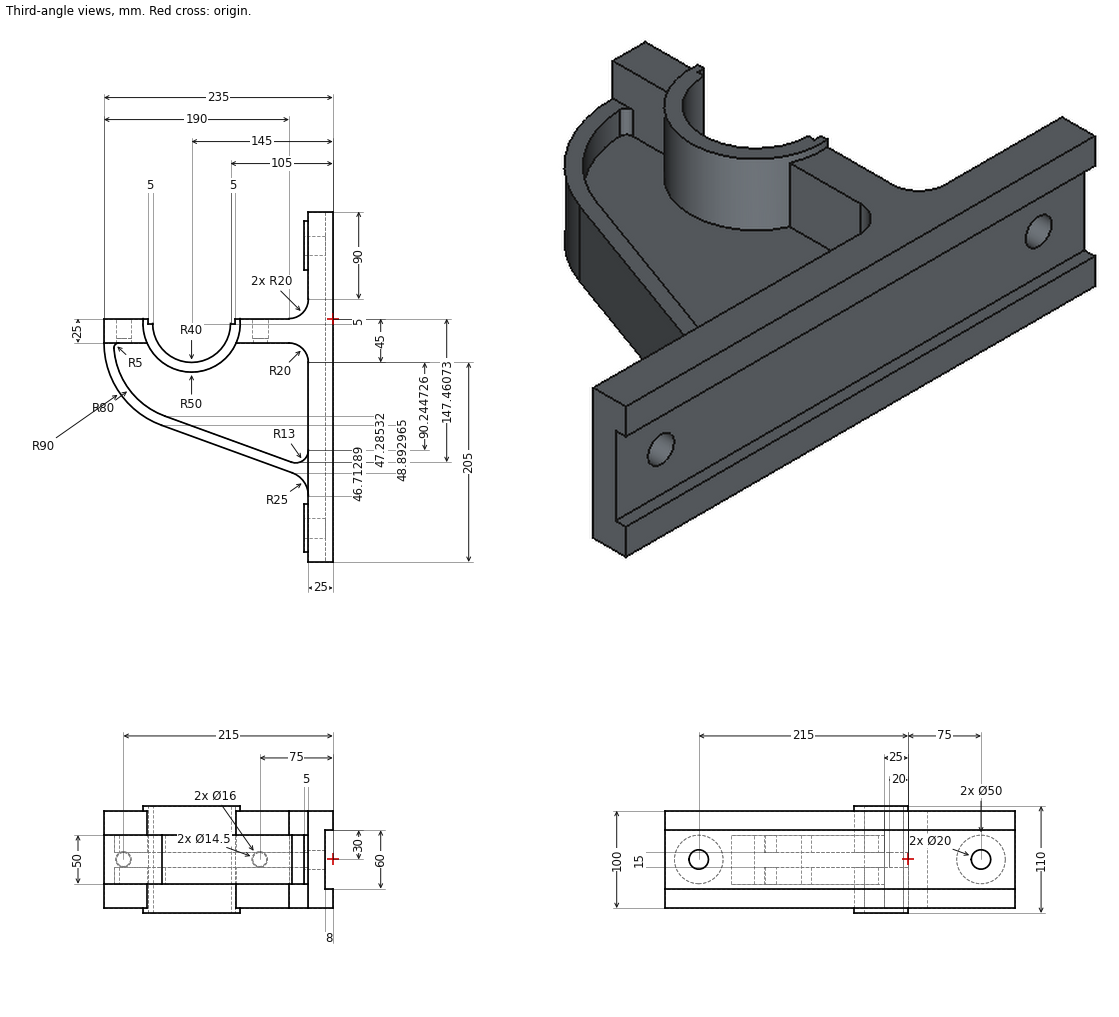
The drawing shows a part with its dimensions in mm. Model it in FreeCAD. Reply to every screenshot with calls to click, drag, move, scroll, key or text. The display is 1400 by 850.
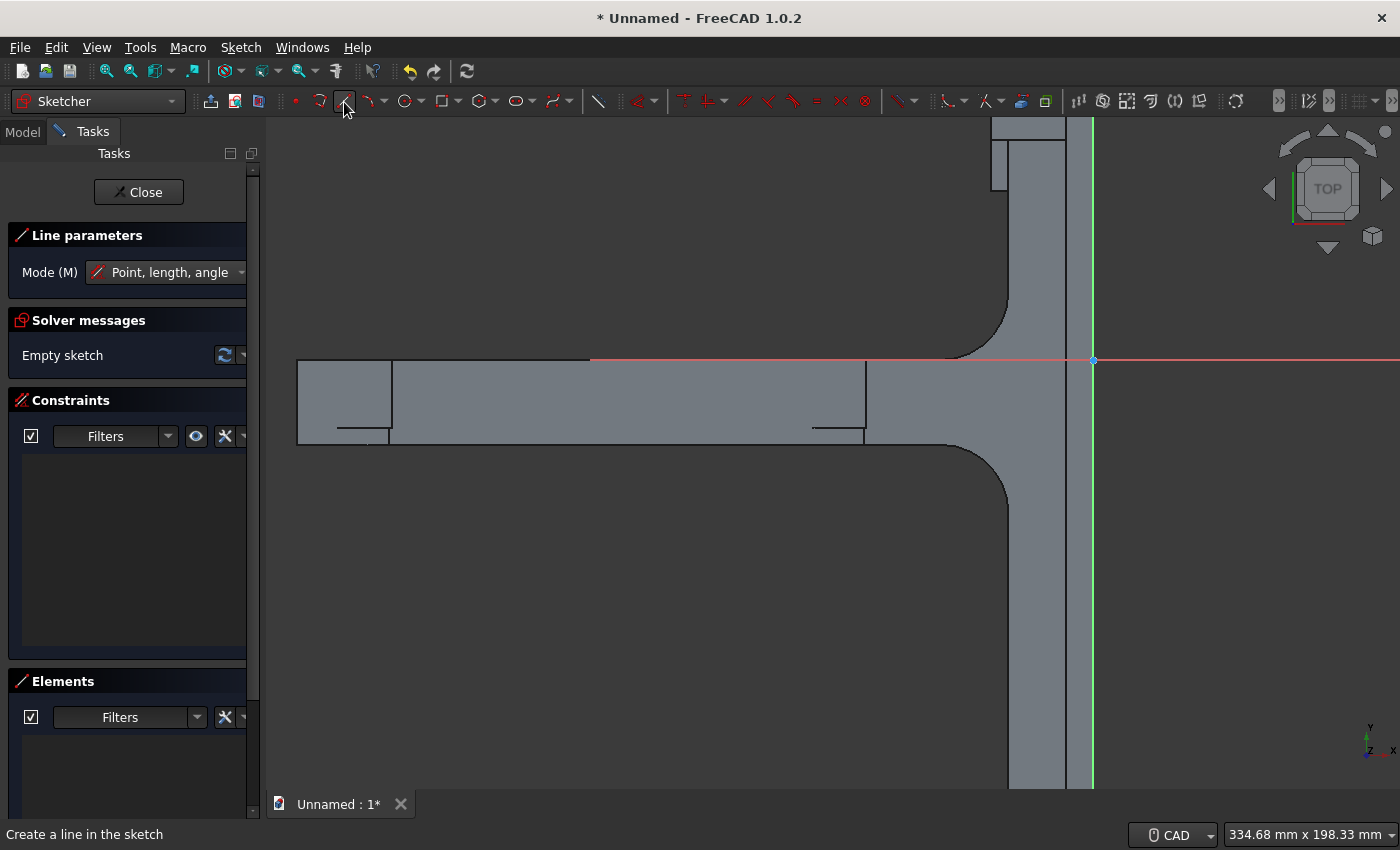
click(770, 360)
click(433, 369)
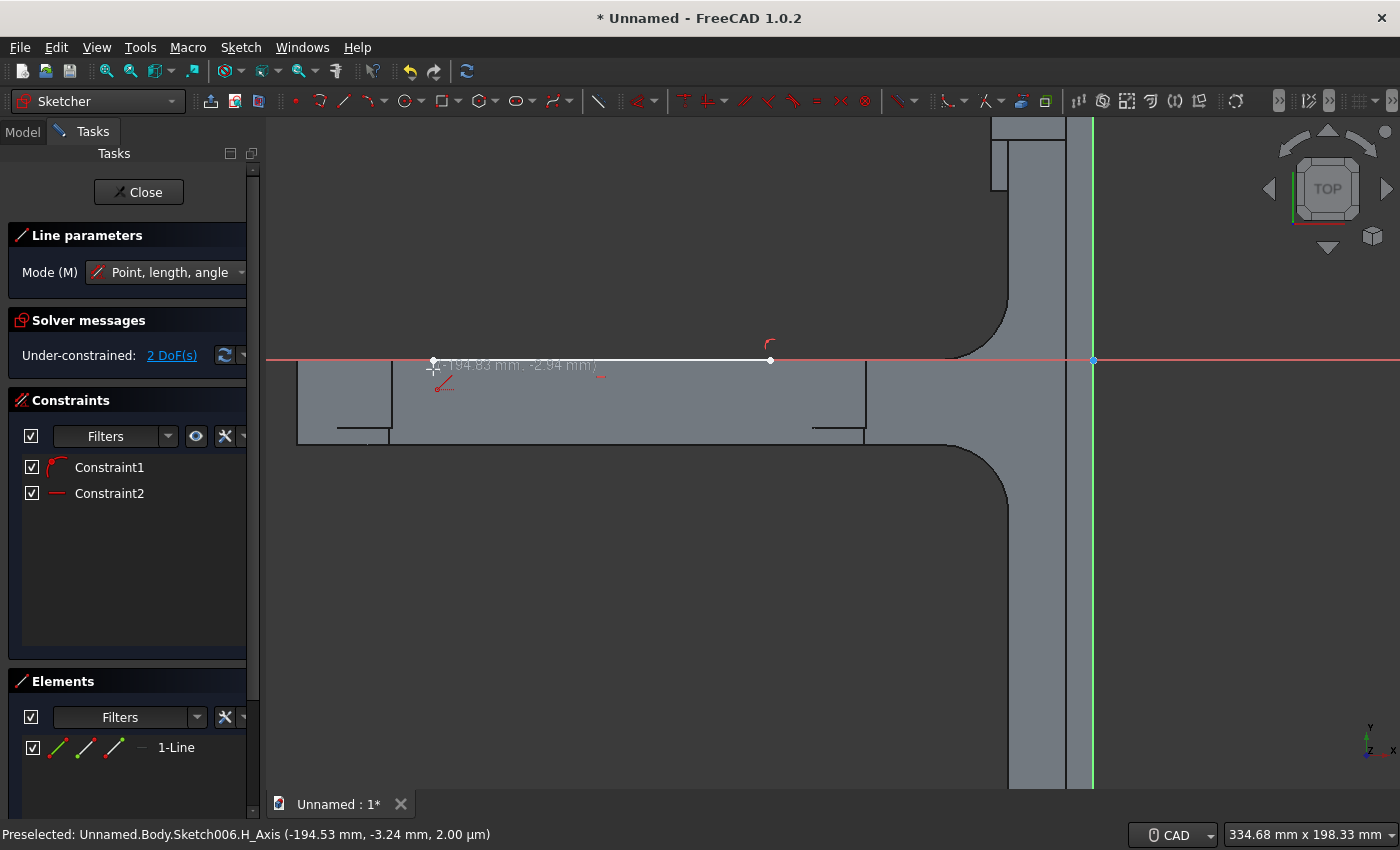
click(368, 102)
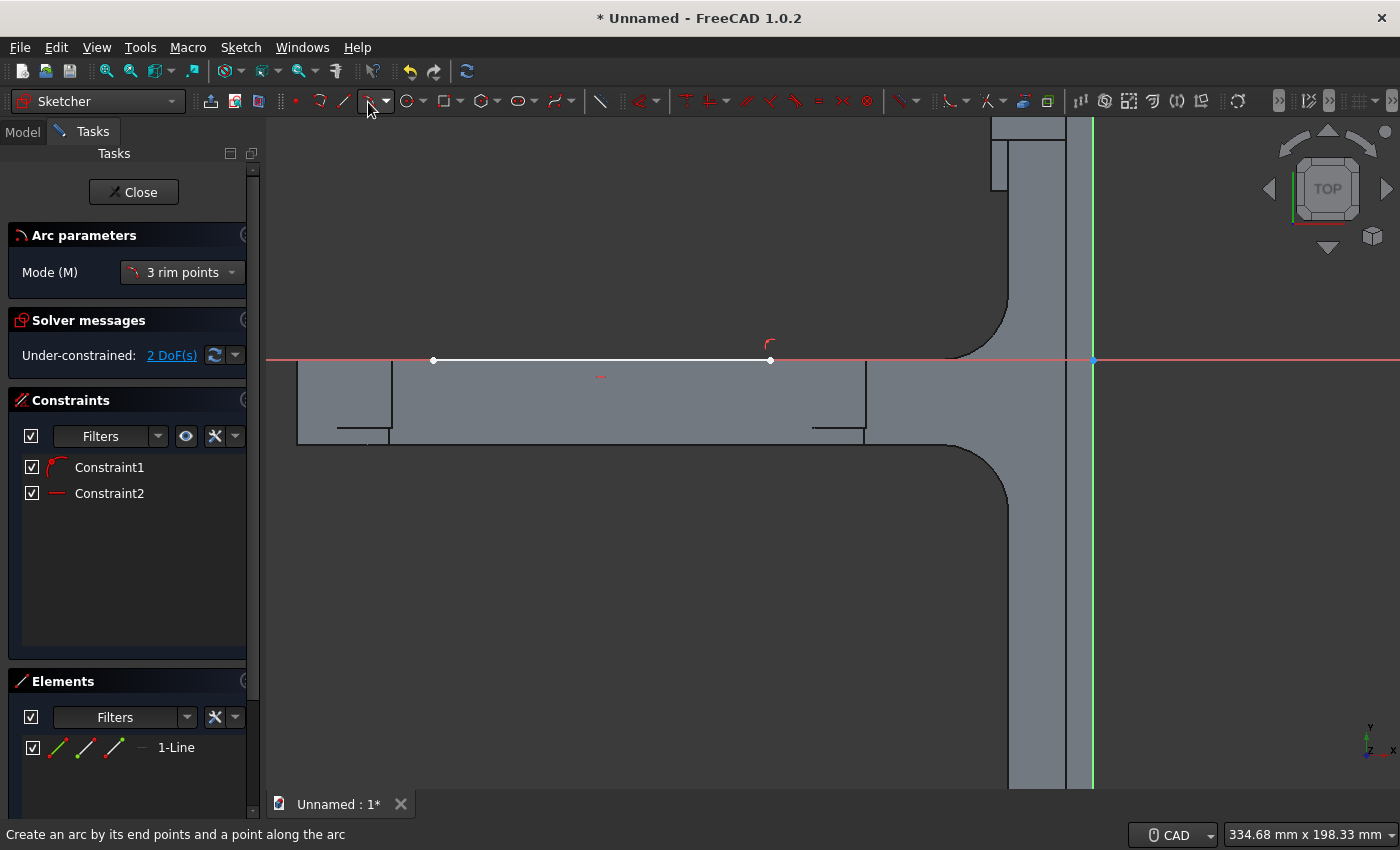
click(433, 360)
click(770, 360)
click(602, 546)
key(Escape)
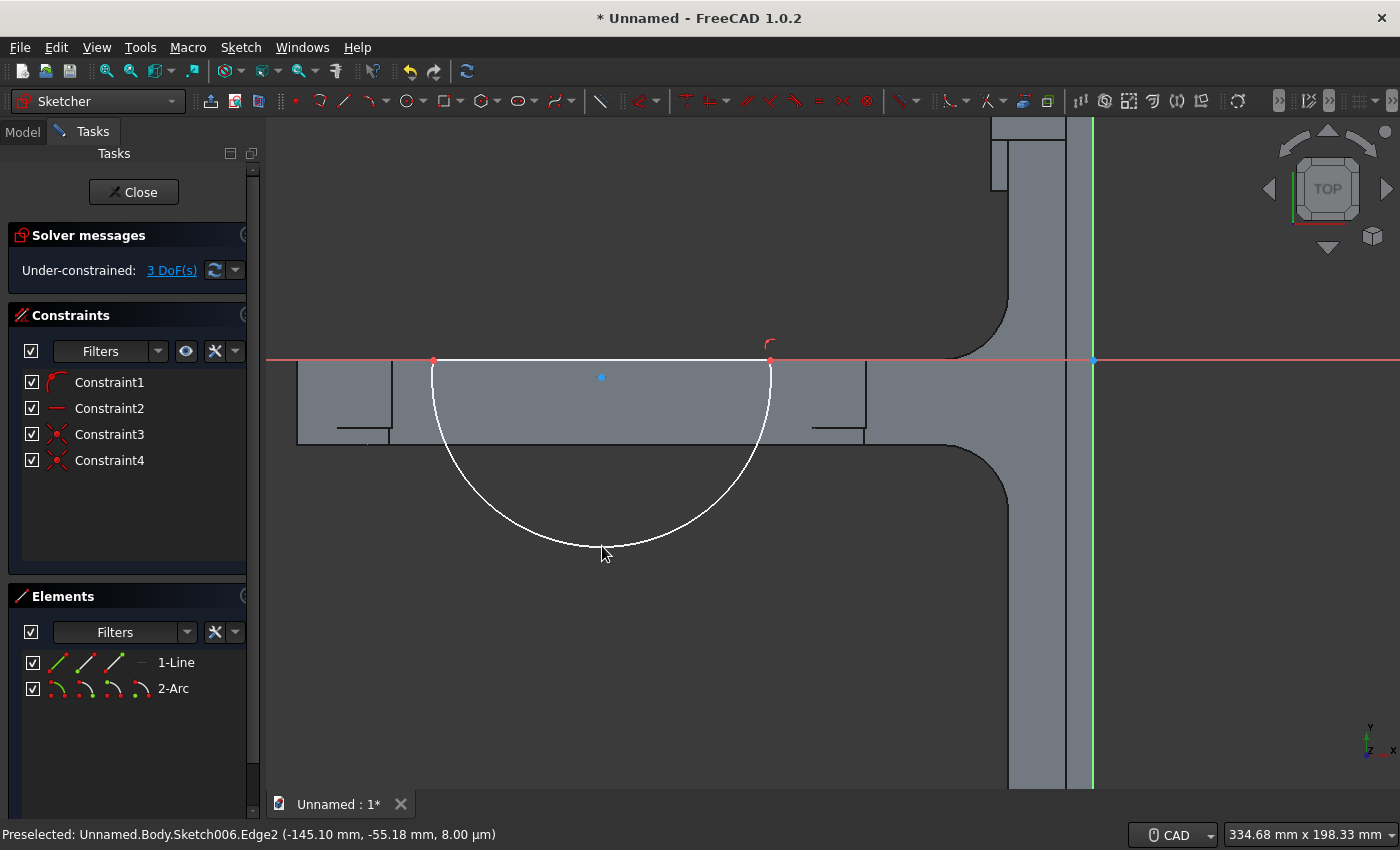
click(640, 102)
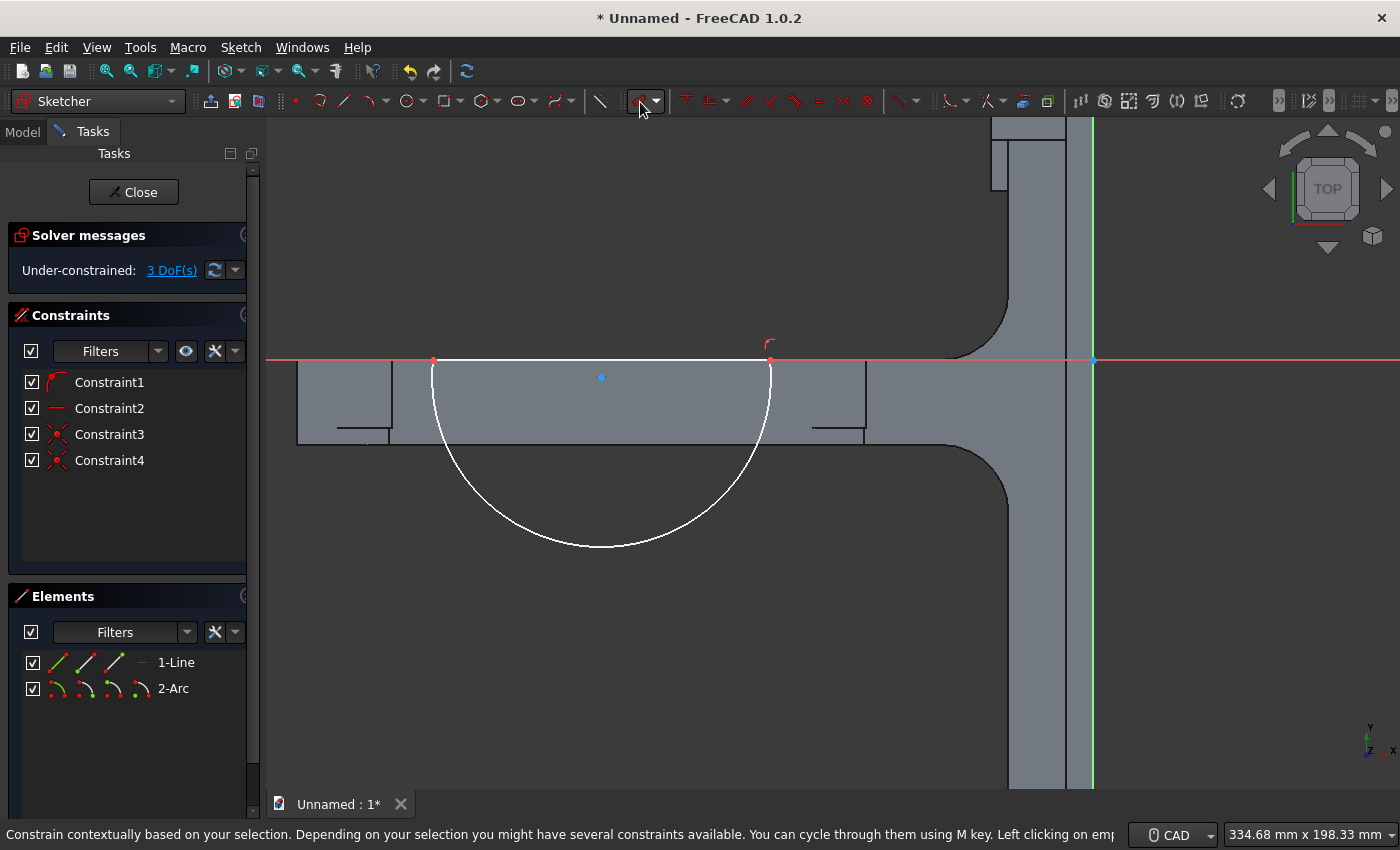
click(496, 510)
click(476, 535)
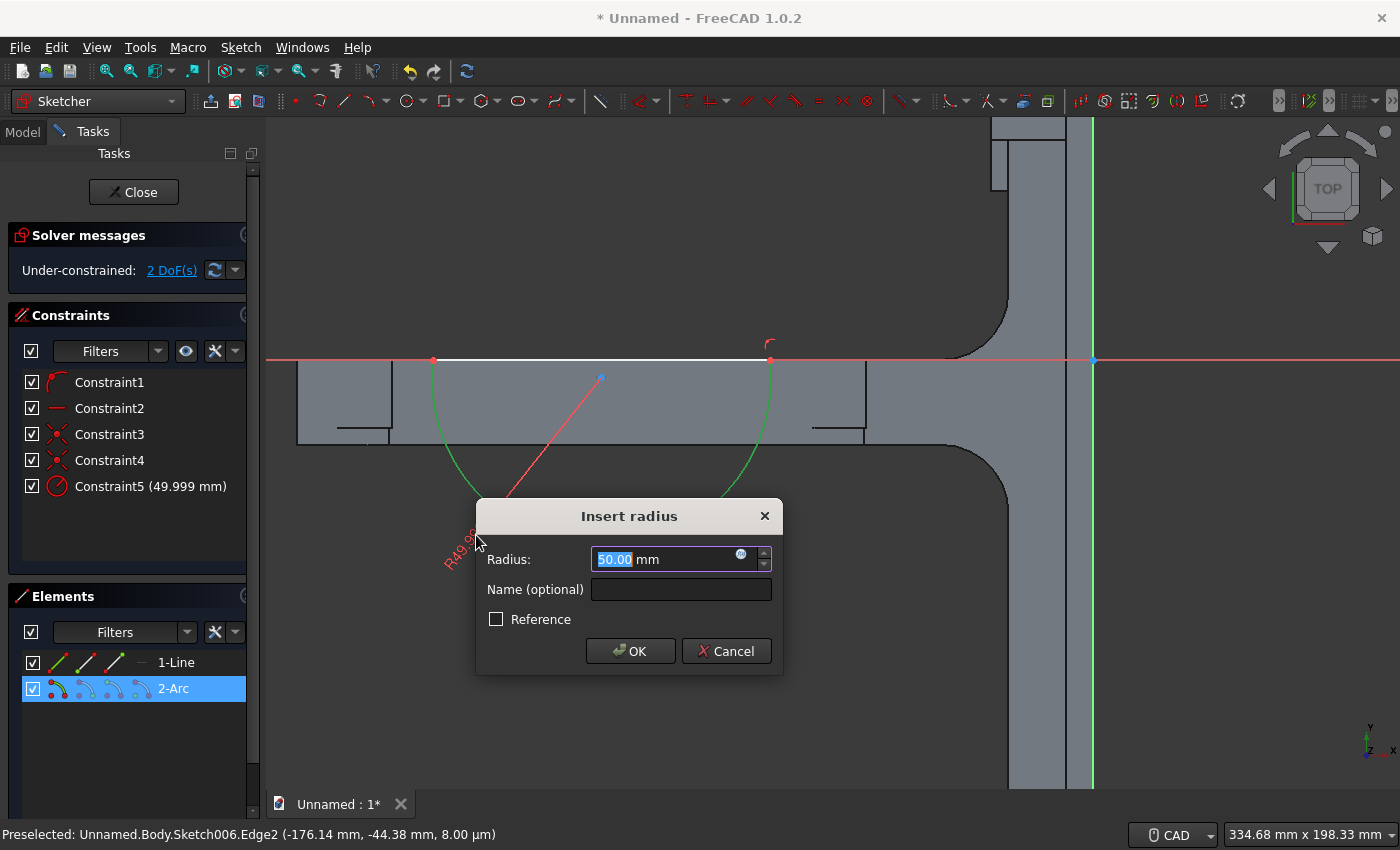
text(50)
key(Return)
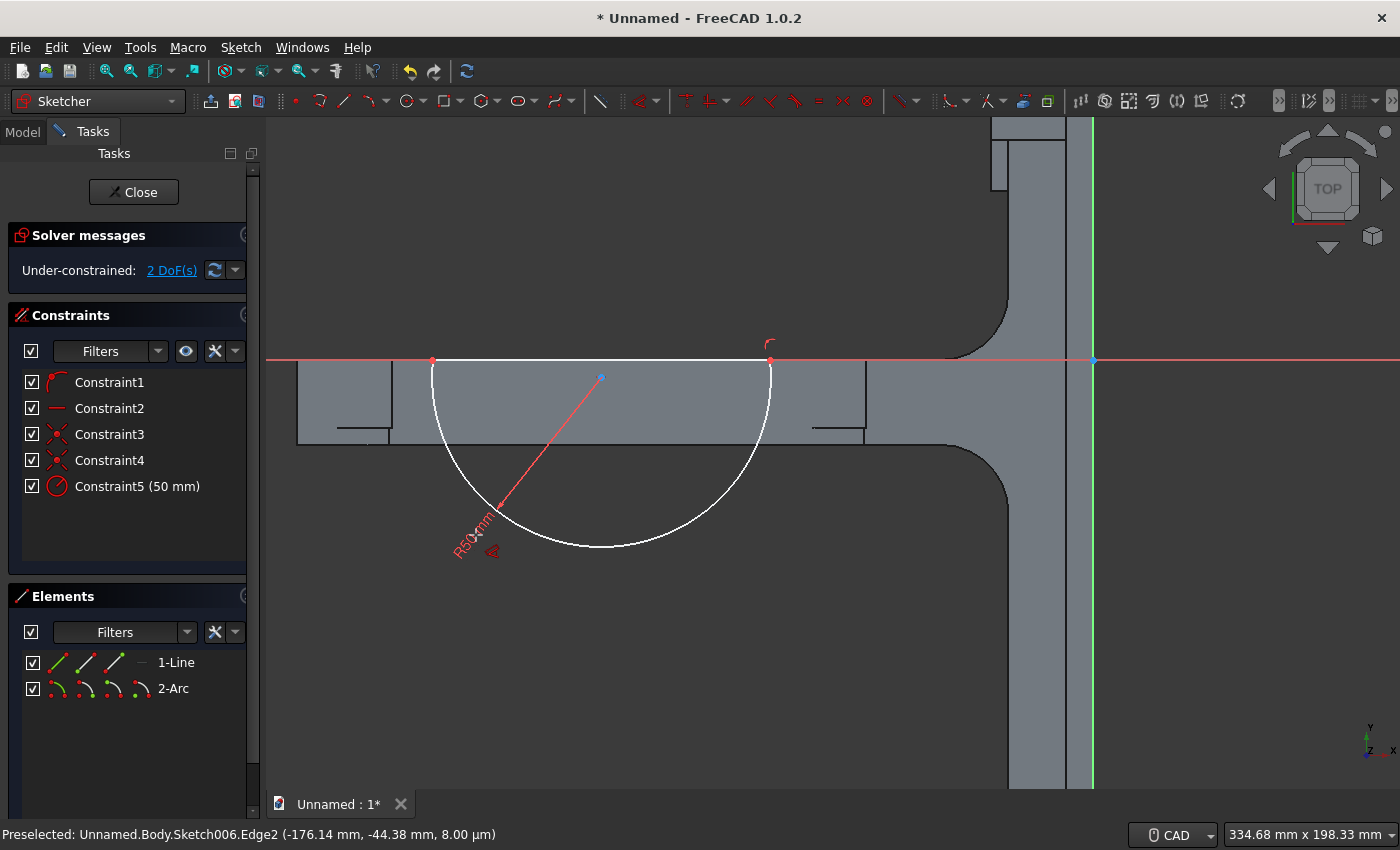
scroll(601, 378, up, 5)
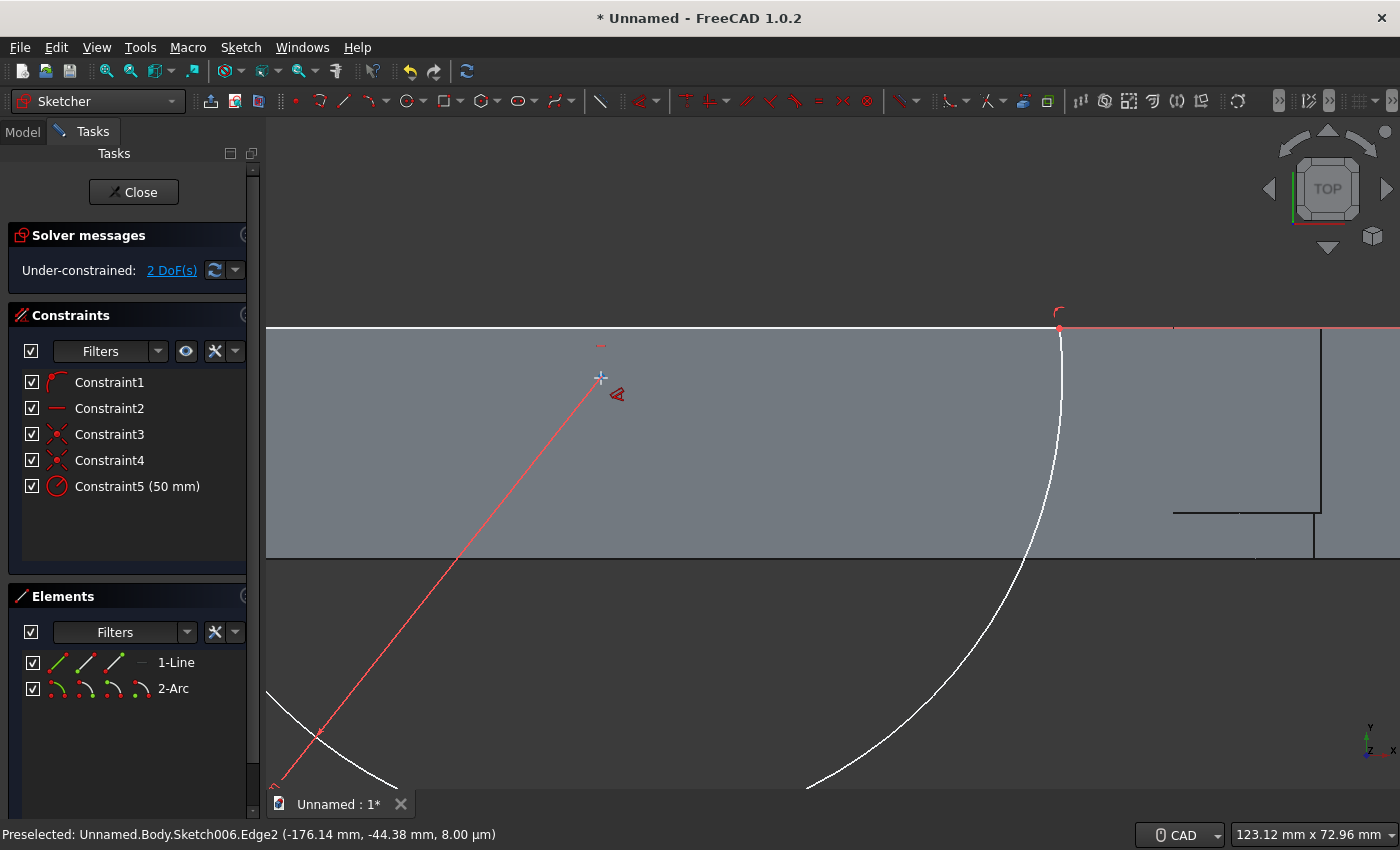
click(602, 376)
click(568, 352)